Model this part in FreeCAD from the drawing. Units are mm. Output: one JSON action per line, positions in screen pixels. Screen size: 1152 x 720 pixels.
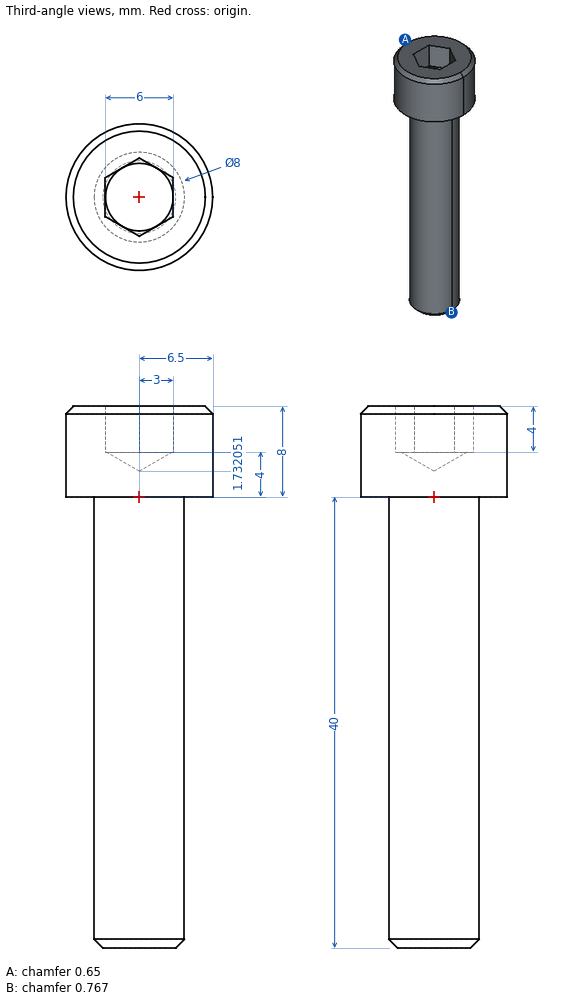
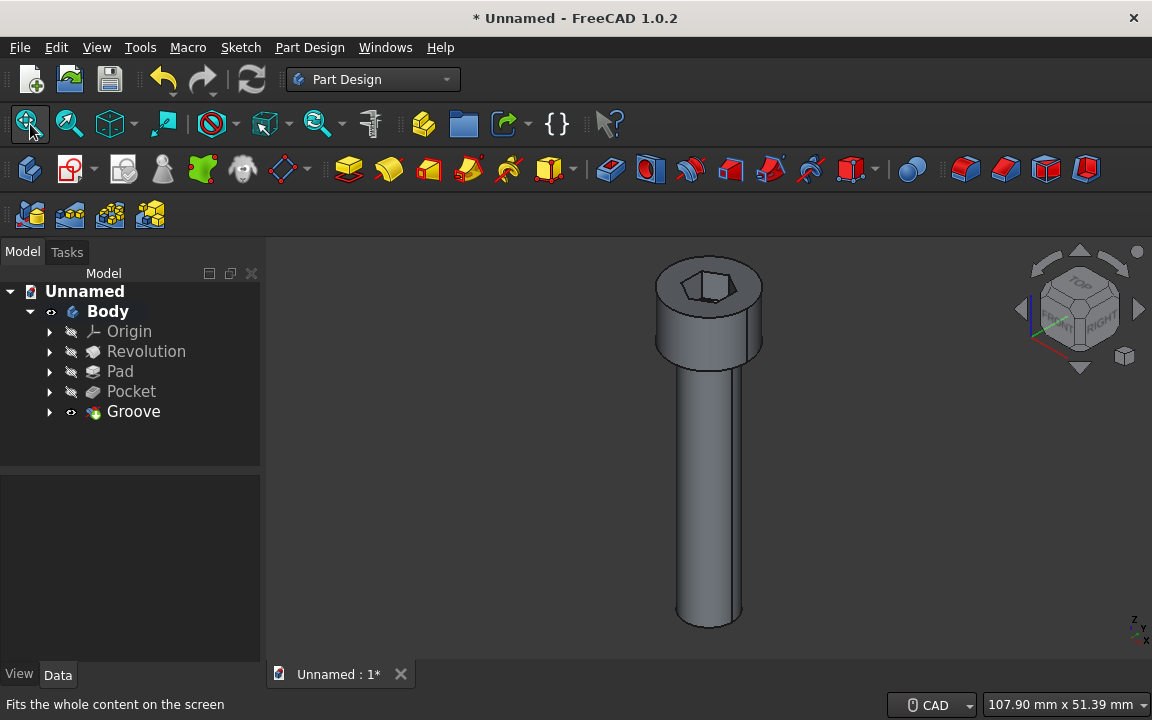
{"action": "left_click", "coordinate": [661, 300]}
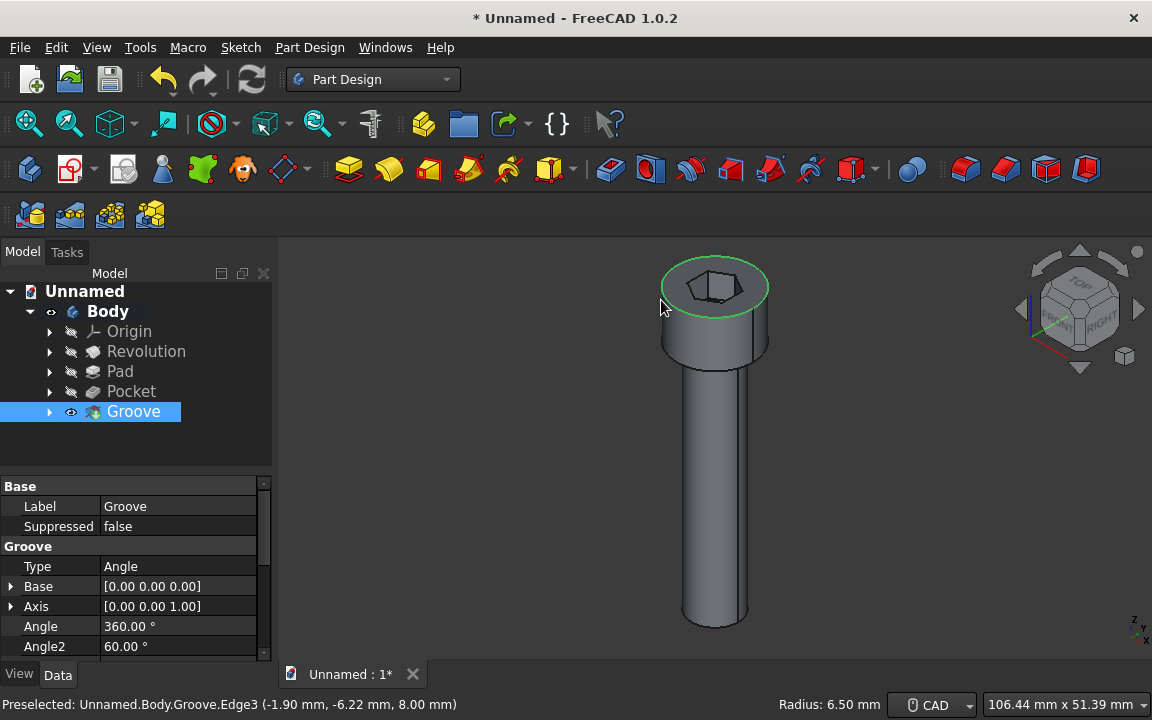
{"action": "left_click", "coordinate": [1006, 170]}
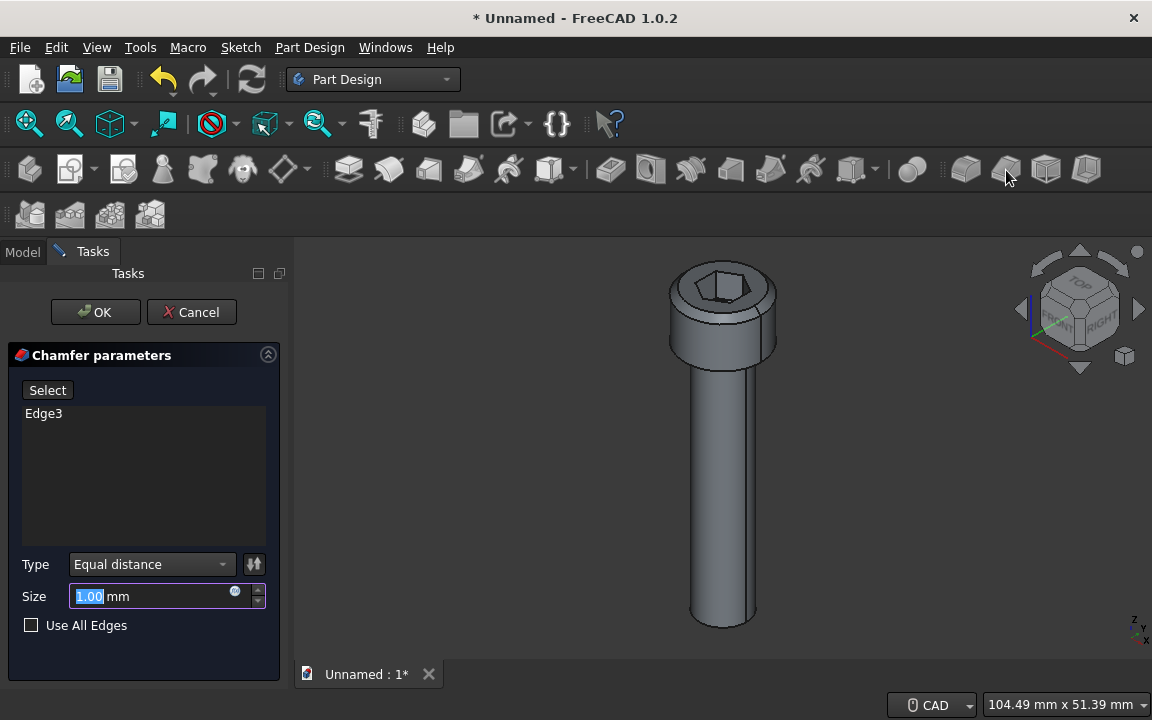
{"action": "type", "text": "0.65"}
{"action": "key", "text": "Tab"}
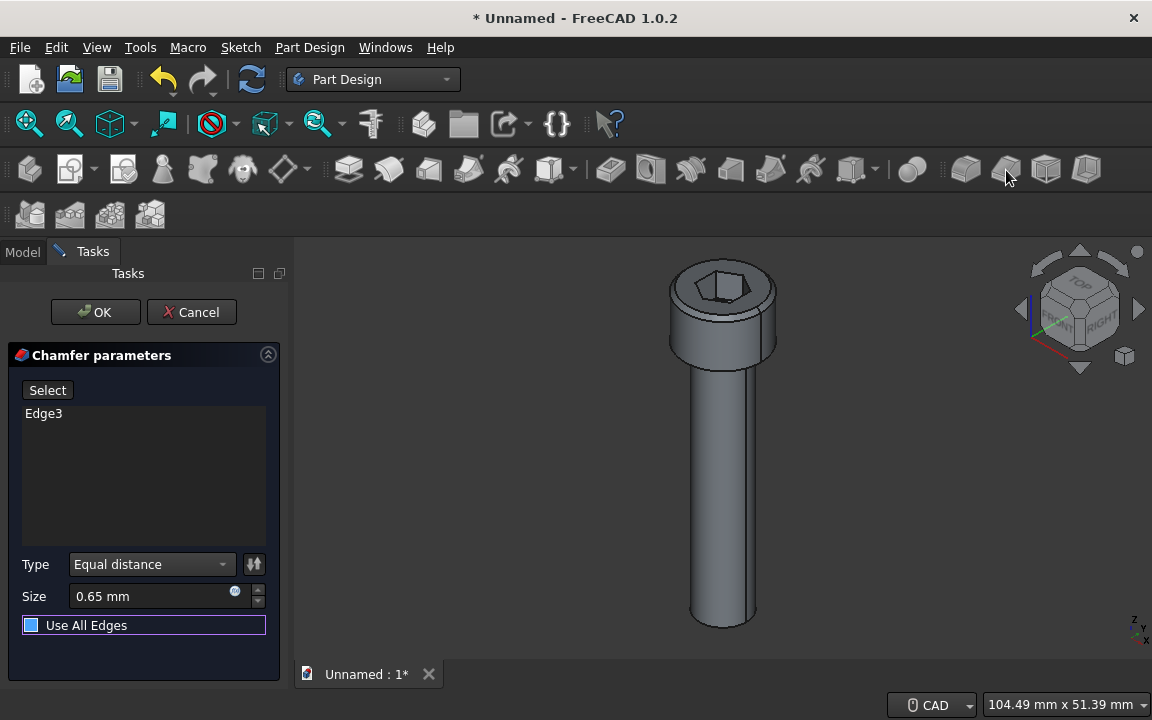
{"action": "left_click", "coordinate": [96, 312]}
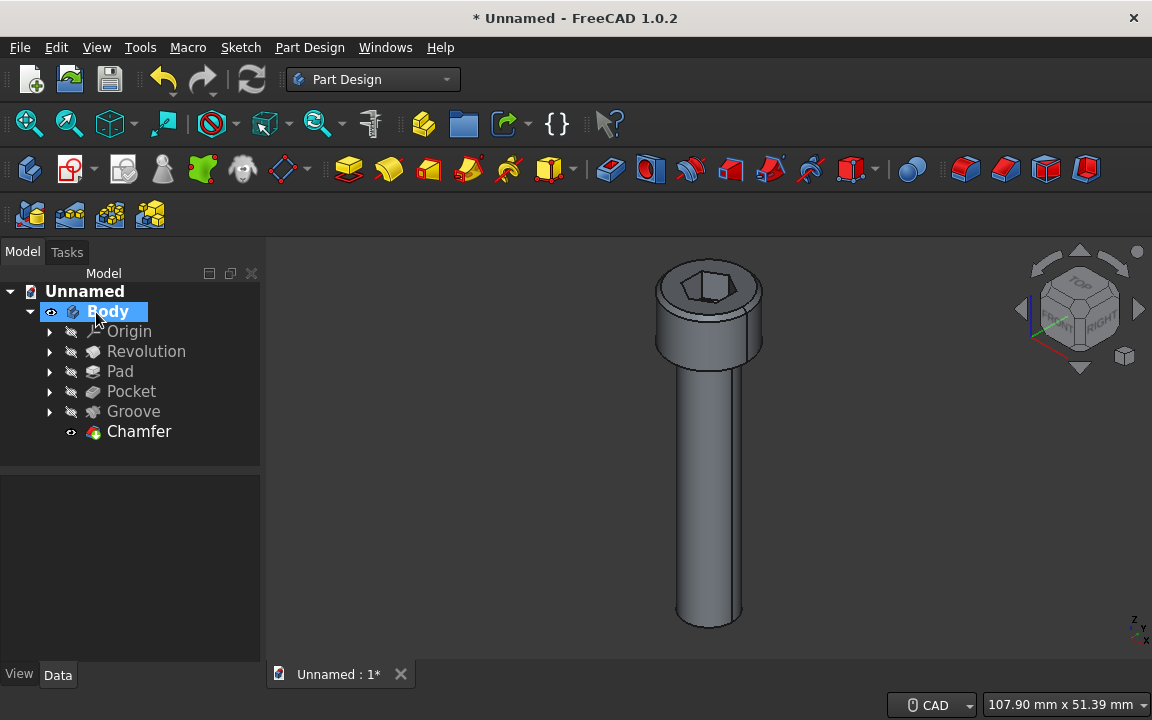
{"action": "key", "text": "2"}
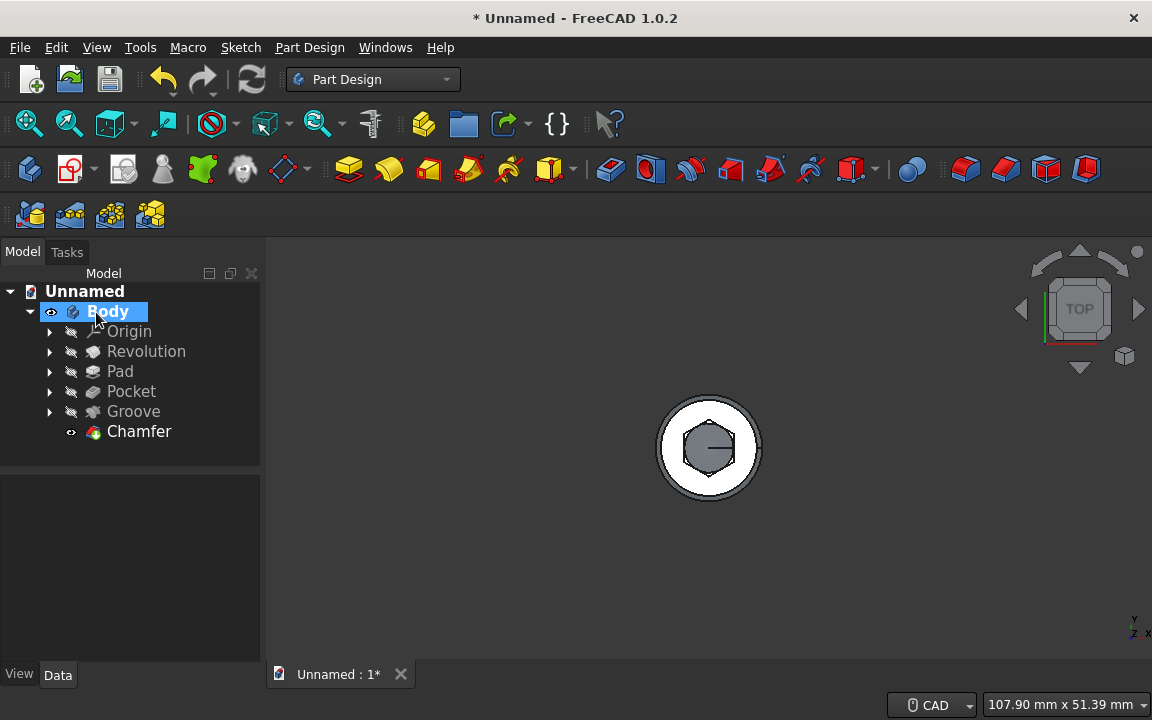
{"action": "left_click", "coordinate": [30, 124]}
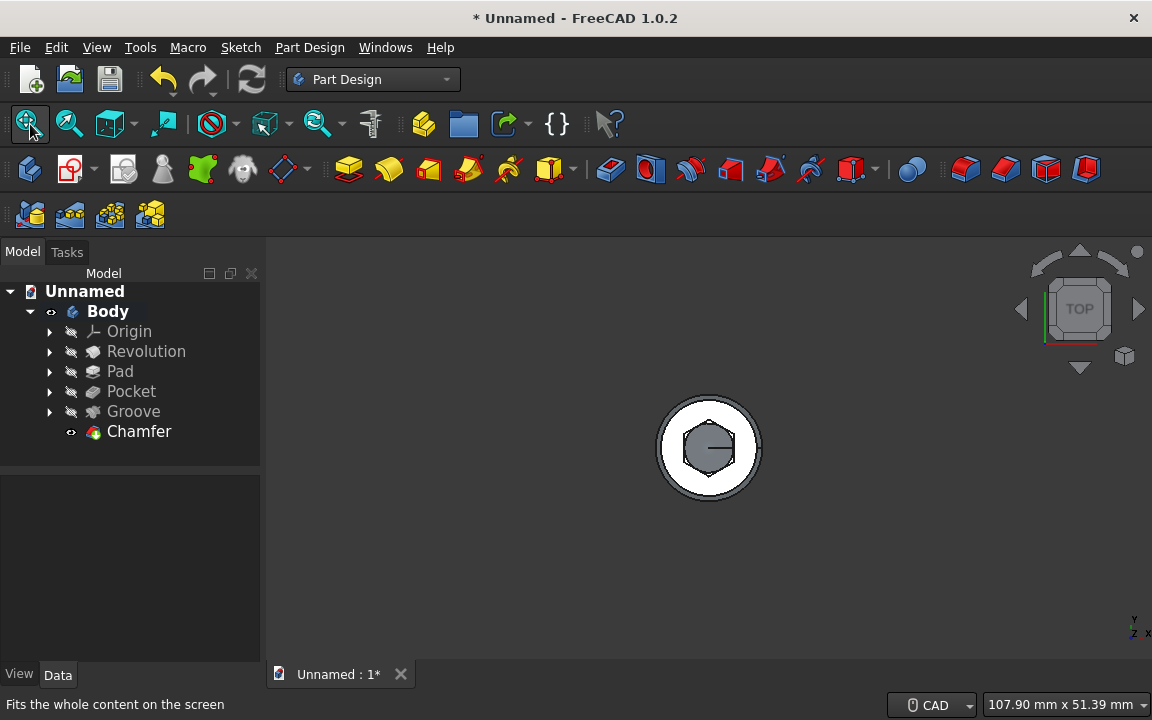
{"action": "key", "text": "0"}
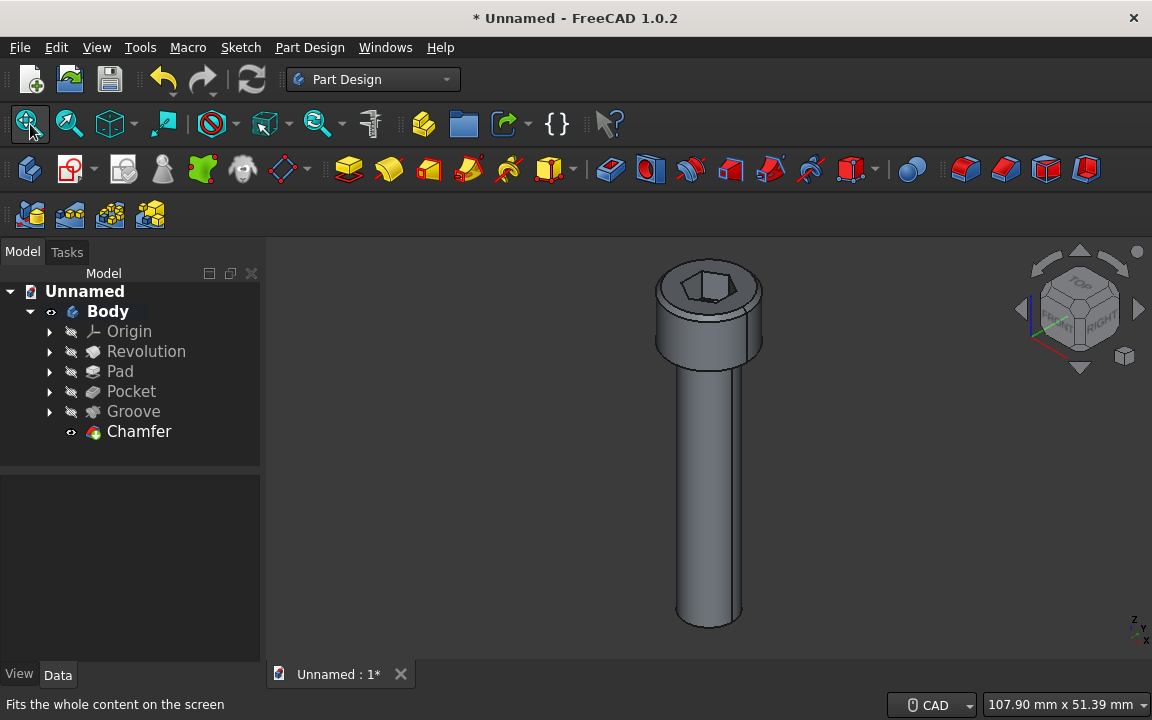
{"action": "key", "text": "1"}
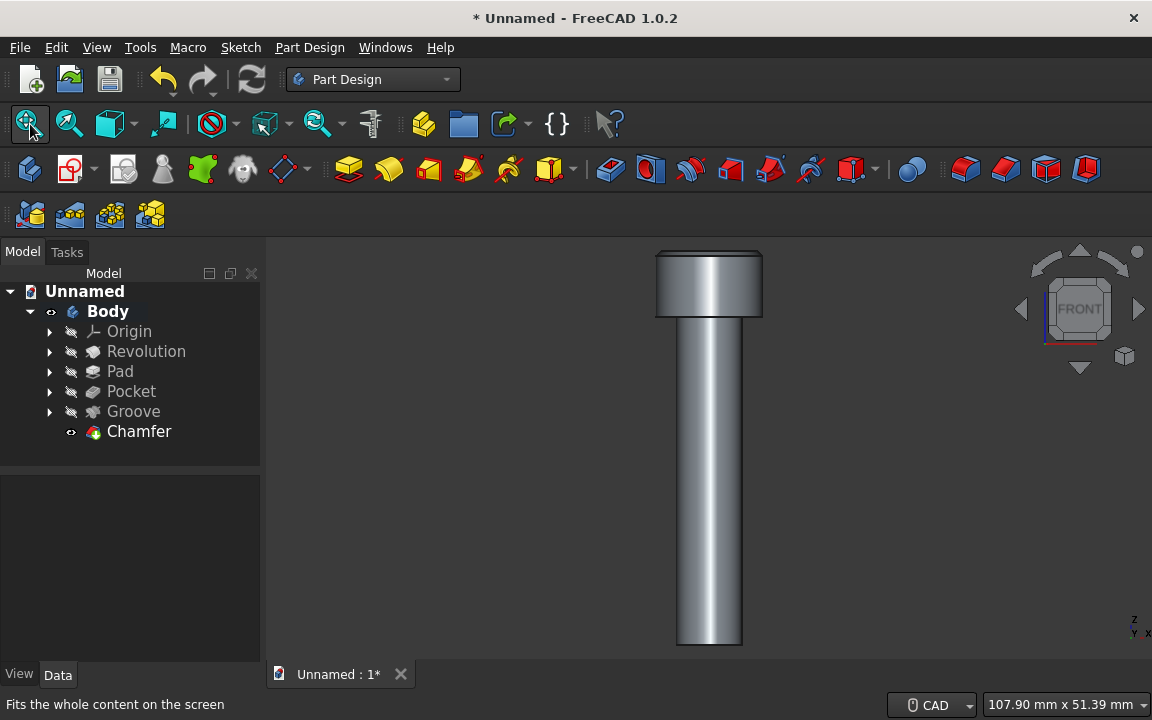
{"action": "key", "text": "3"}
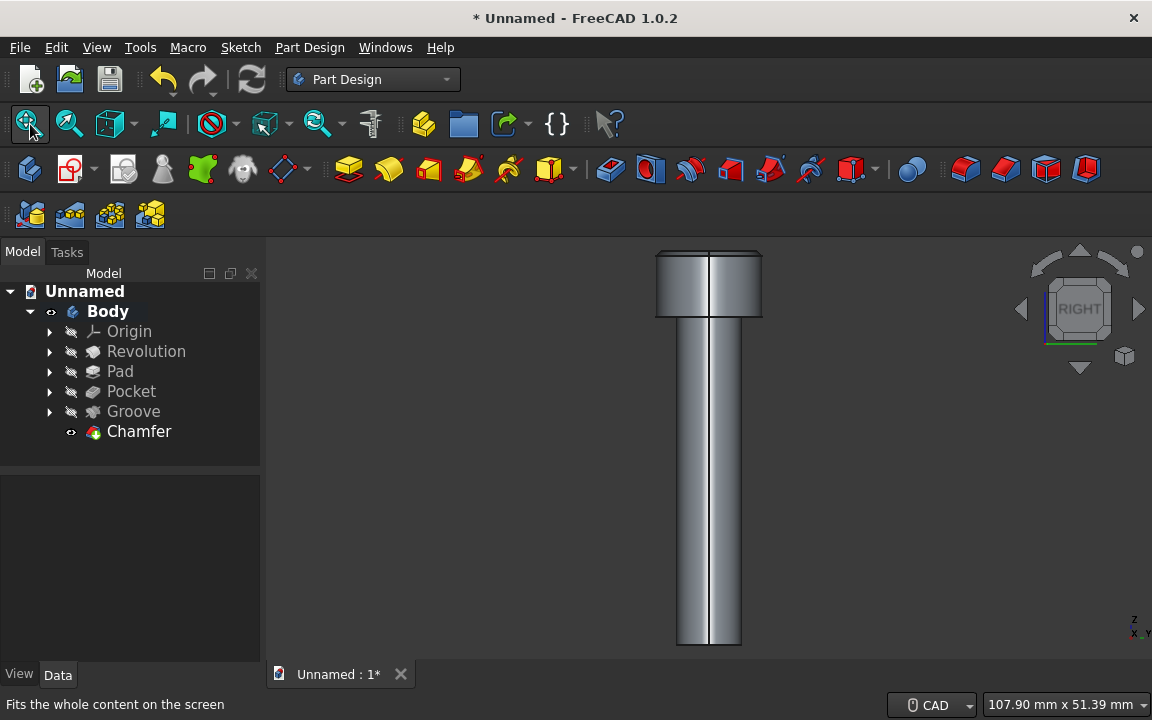
{"action": "key", "text": "5"}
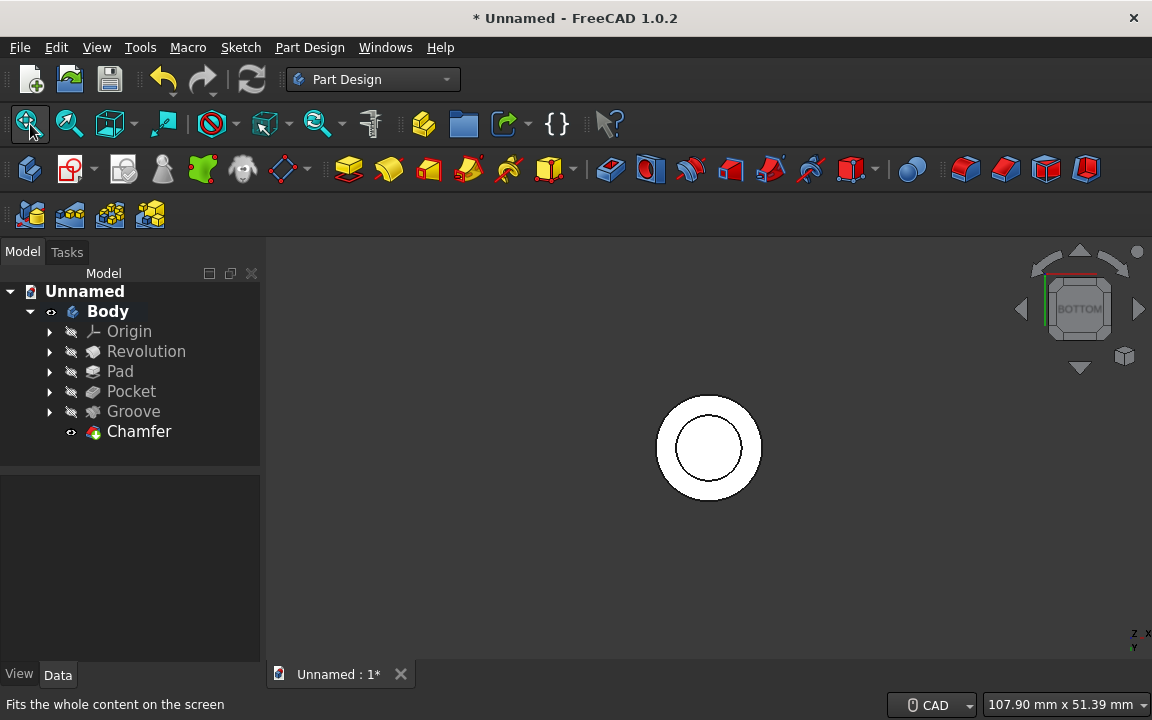
{"action": "left_click", "coordinate": [30, 124]}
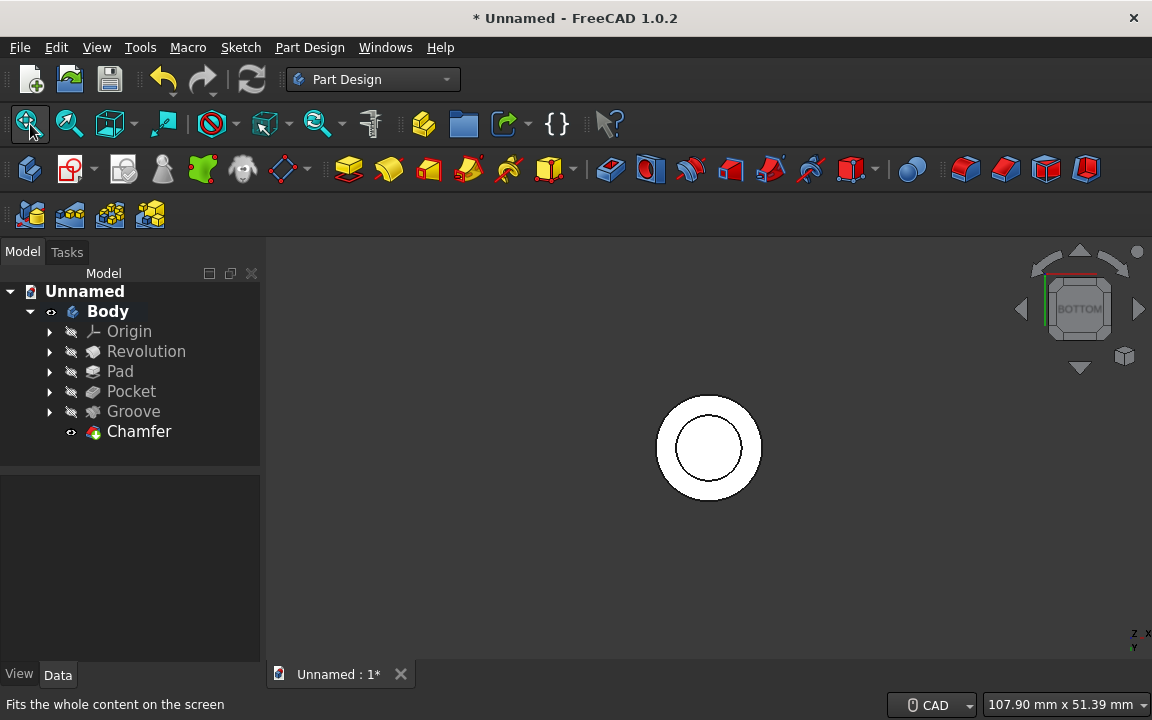
{"action": "left_click", "coordinate": [676, 447]}